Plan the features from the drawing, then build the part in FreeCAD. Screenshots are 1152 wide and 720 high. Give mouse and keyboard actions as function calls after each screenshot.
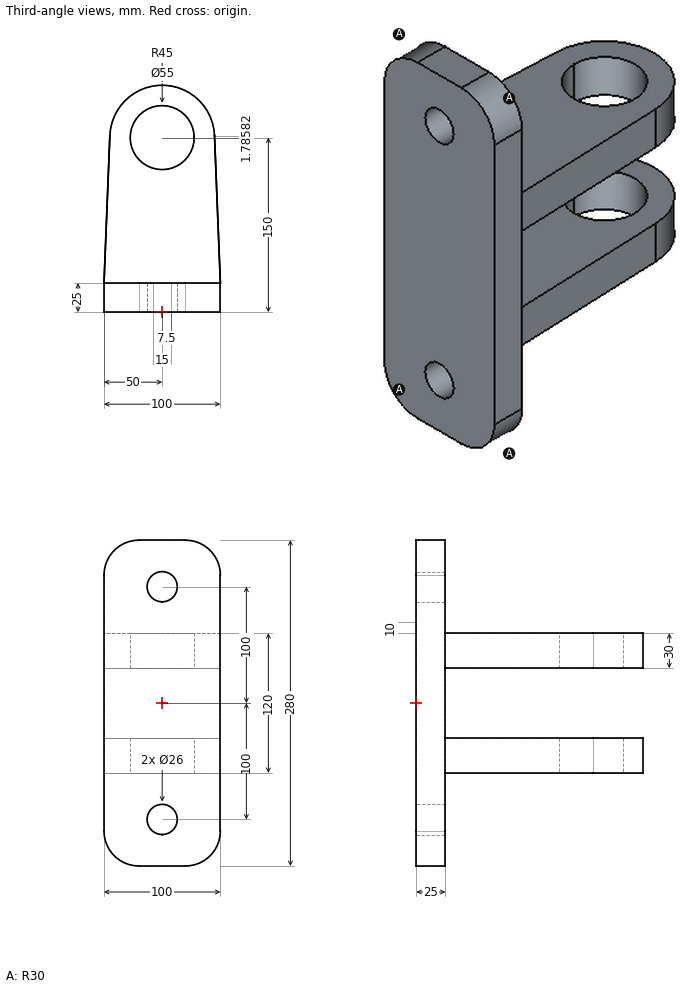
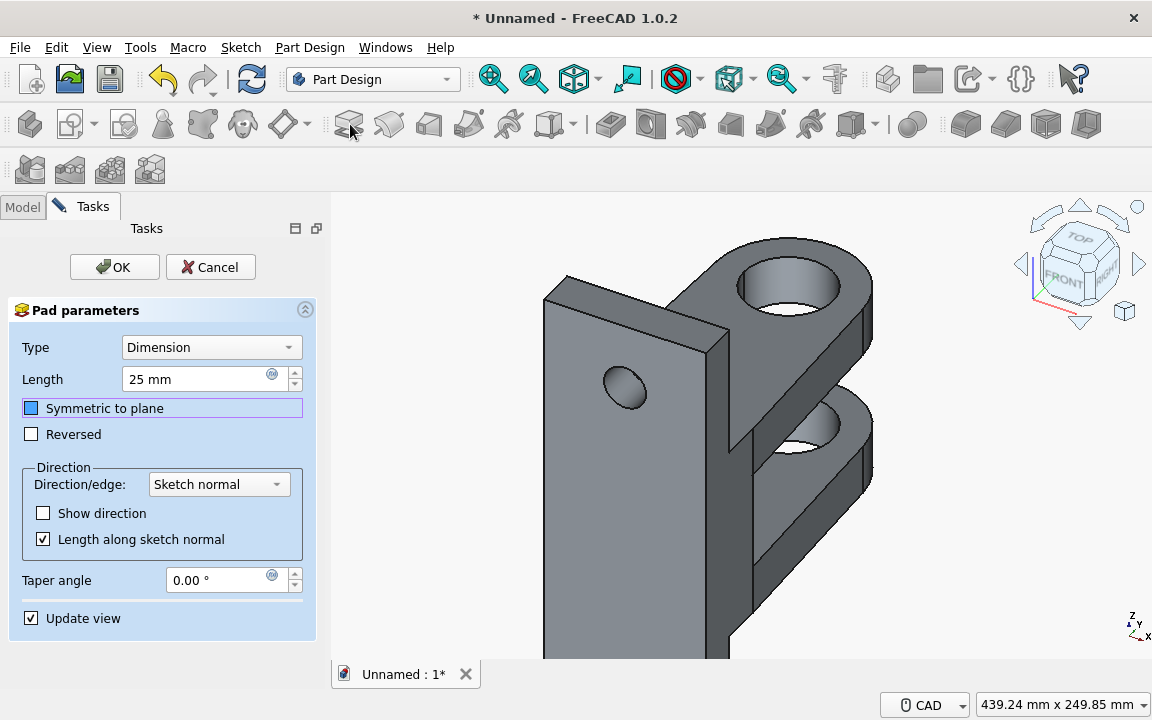
click(30, 434)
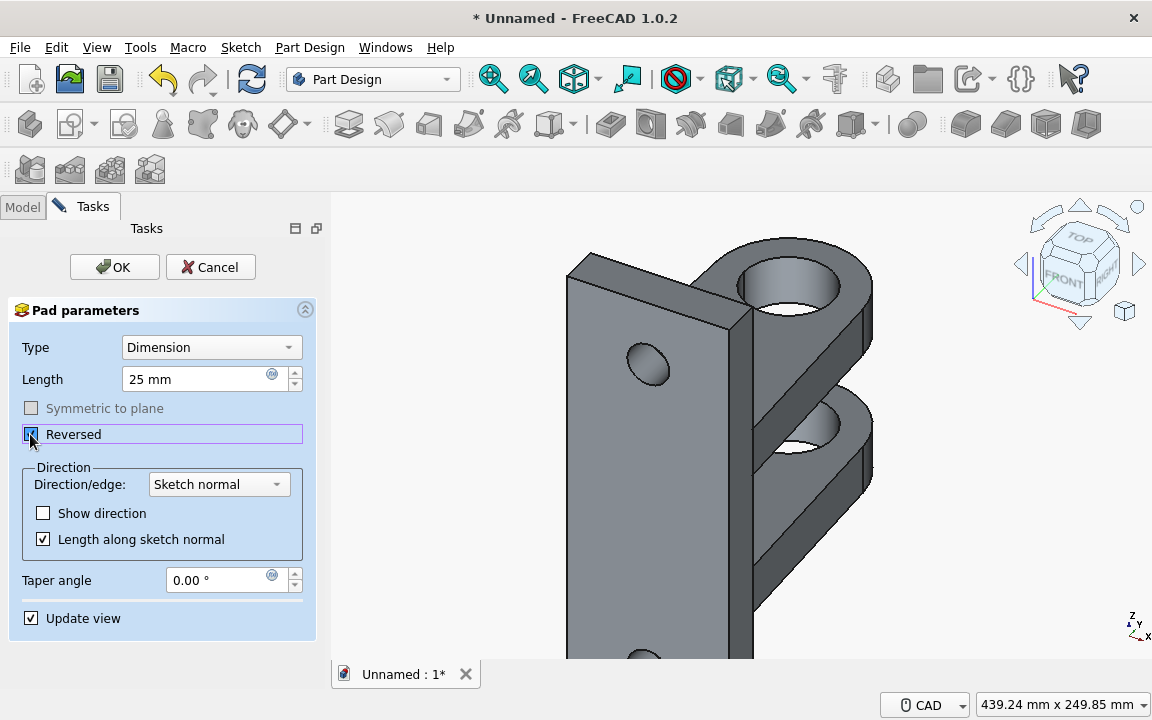
click(115, 267)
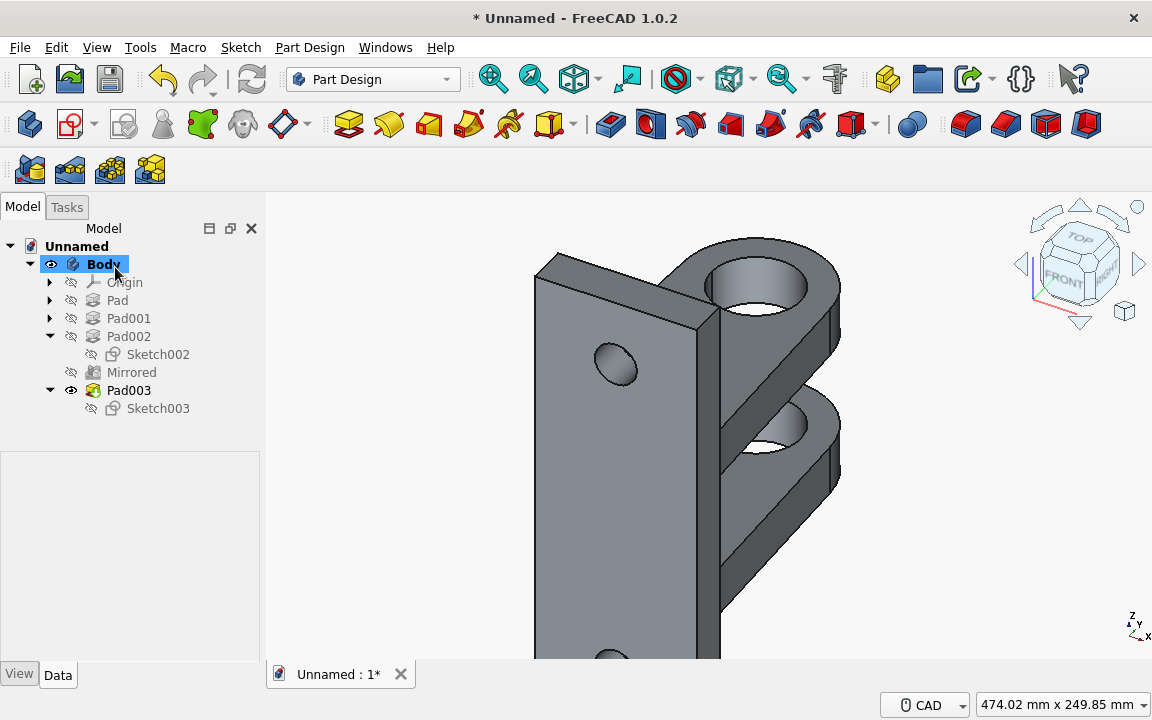
click(494, 80)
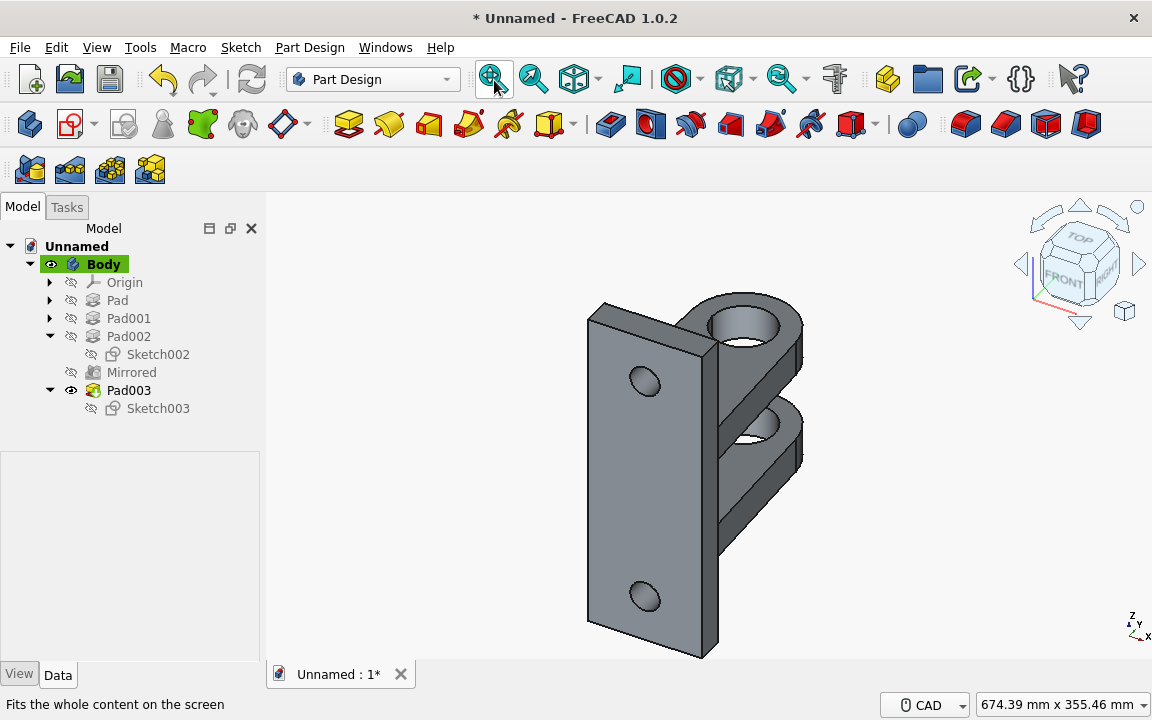
click(710, 348)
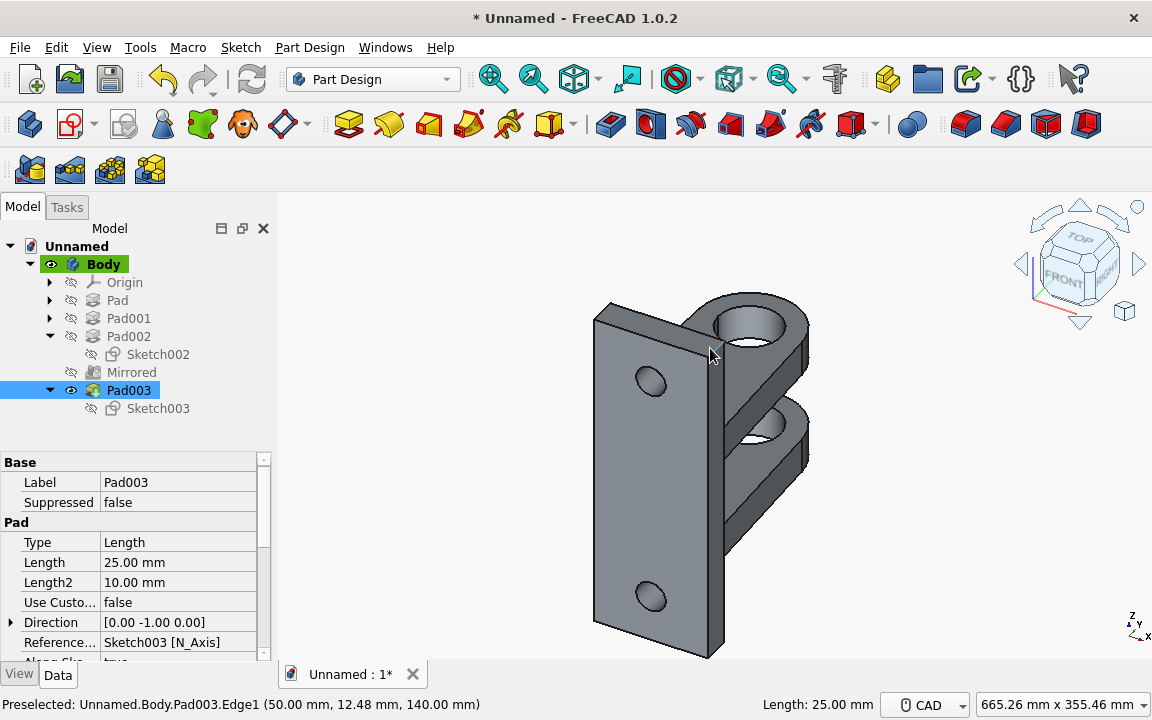
key(0)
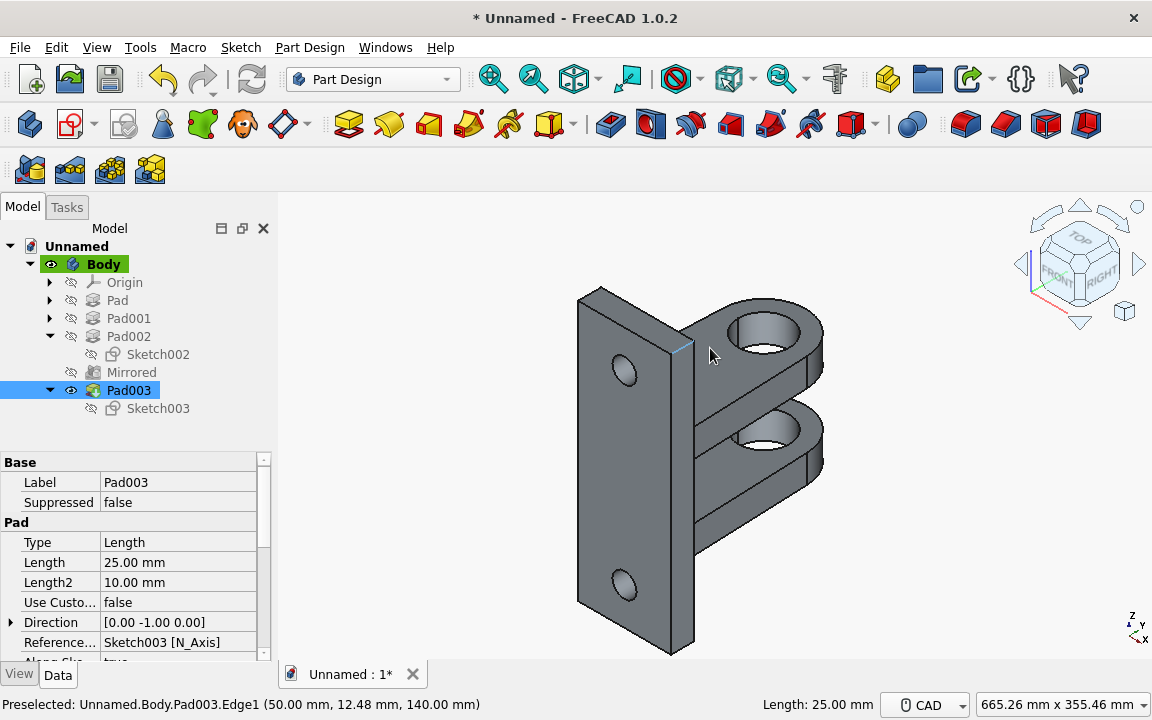
key(2)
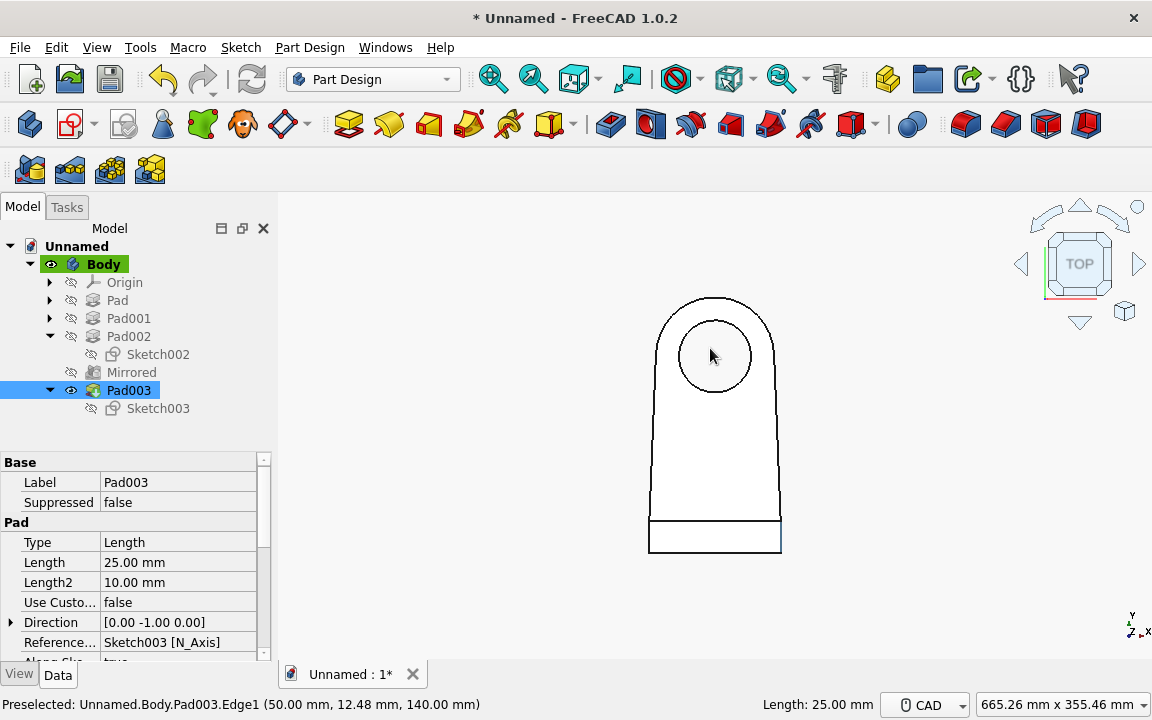
click(649, 536, ctrl)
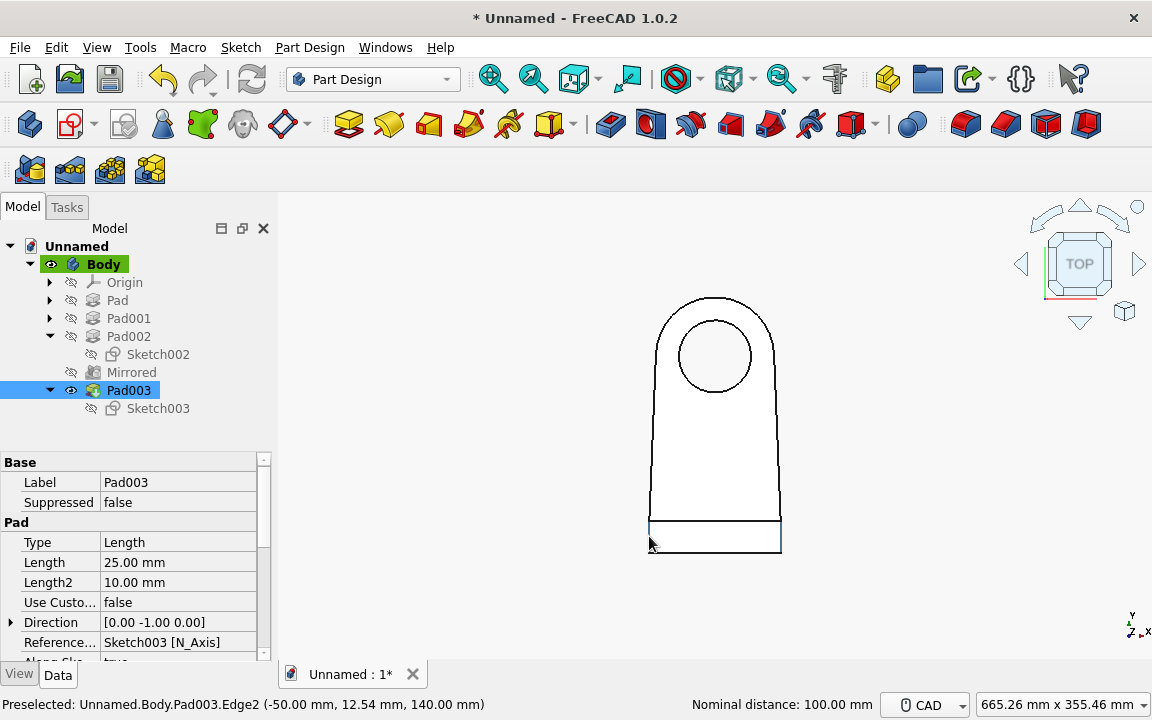
key(1)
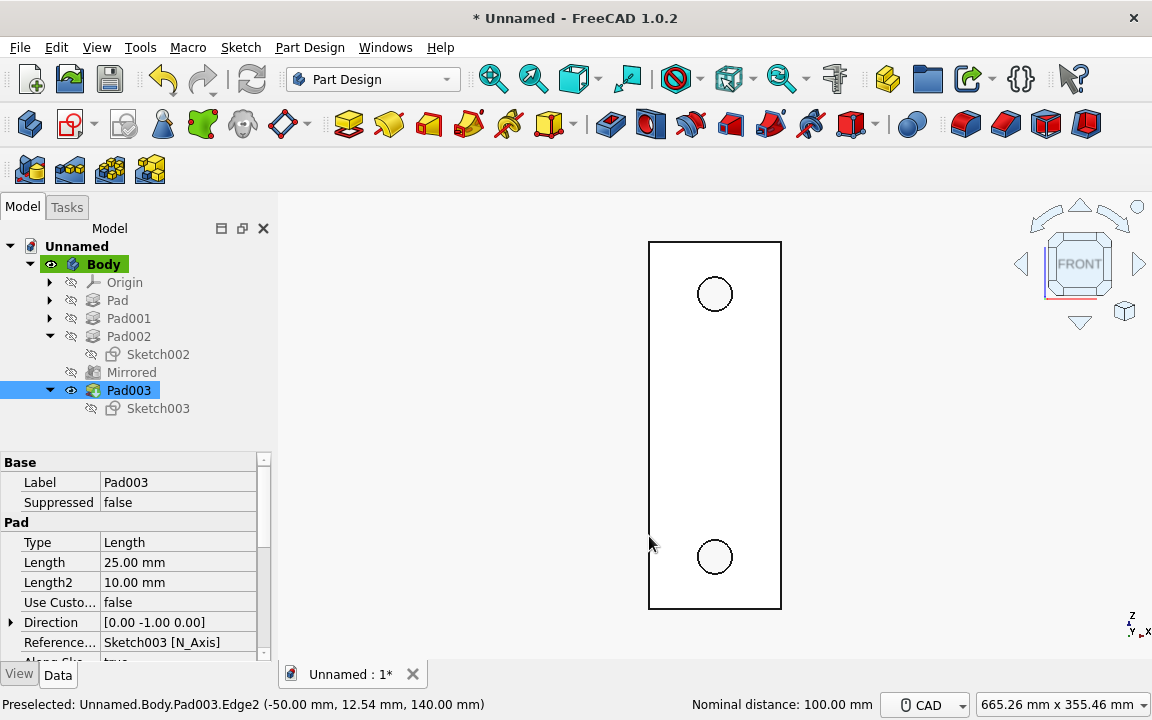
key(3)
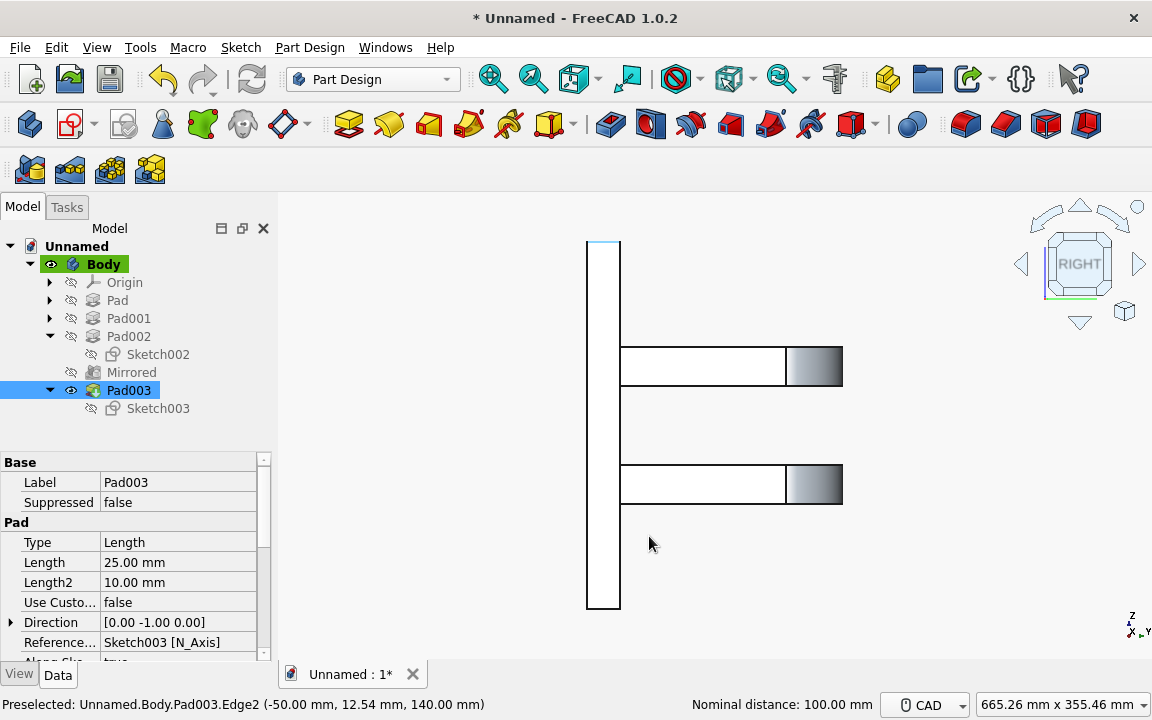
click(603, 608, ctrl)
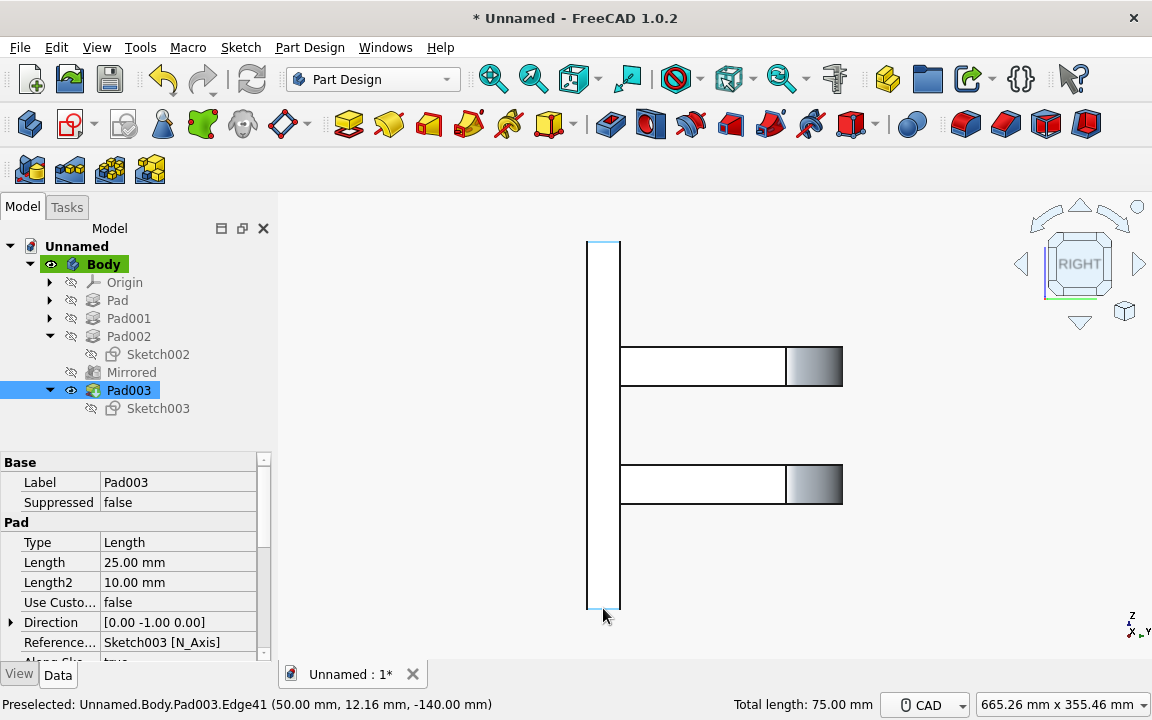
key(5)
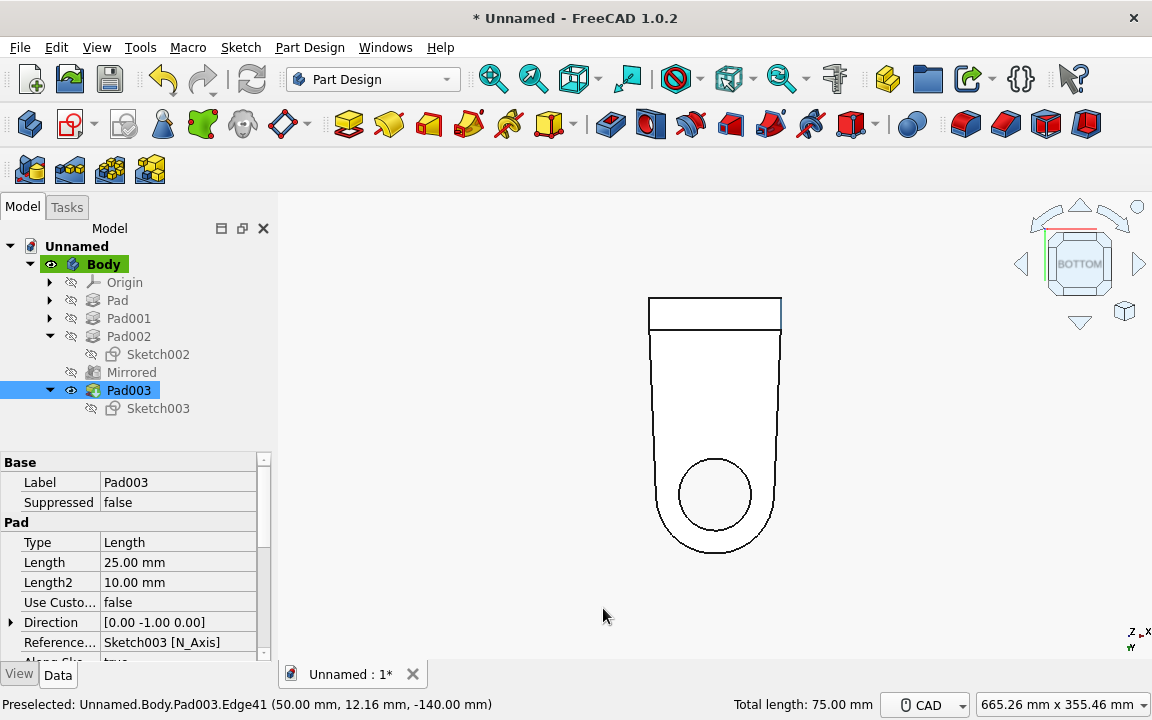
click(649, 313, ctrl)